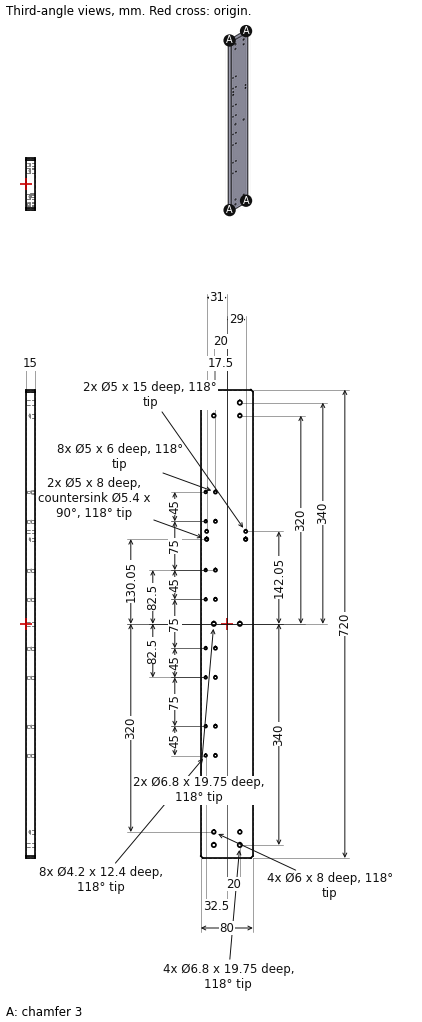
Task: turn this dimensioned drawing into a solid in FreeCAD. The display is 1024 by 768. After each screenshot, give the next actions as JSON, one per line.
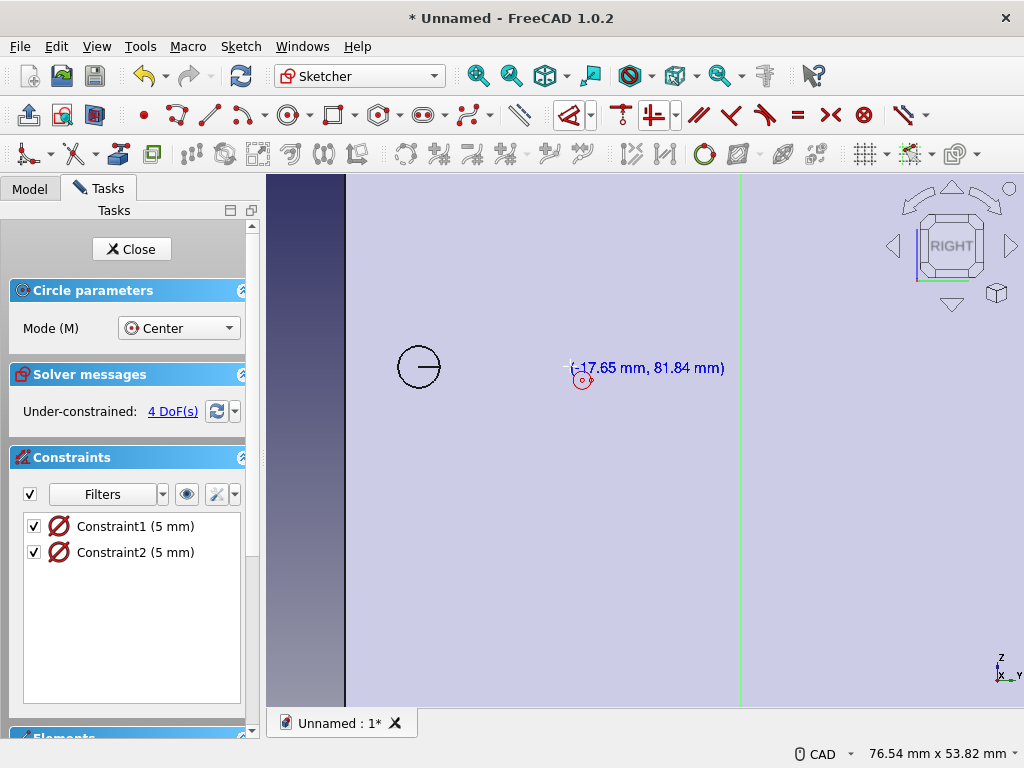
{"action": "scroll", "coordinate": [570, 366], "scroll_direction": "down", "scroll_amount": 12}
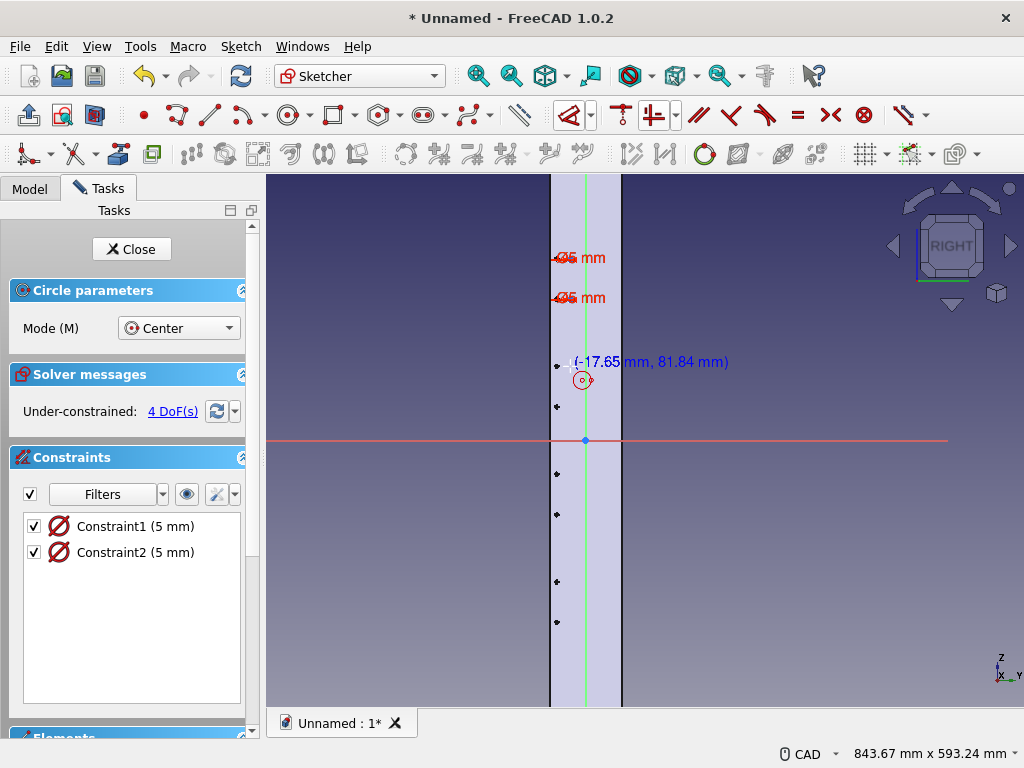
{"action": "left_click", "coordinate": [570, 366]}
{"action": "mouse_move", "coordinate": [572, 365]}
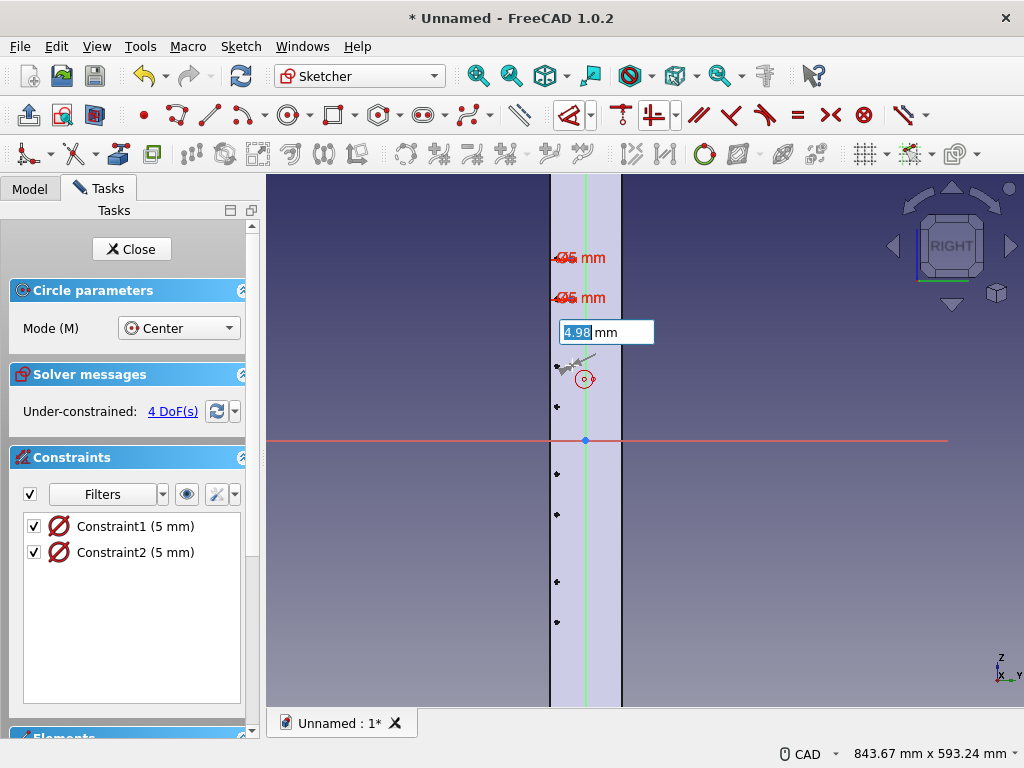
{"action": "type", "text": "5"}
{"action": "key", "text": "Return"}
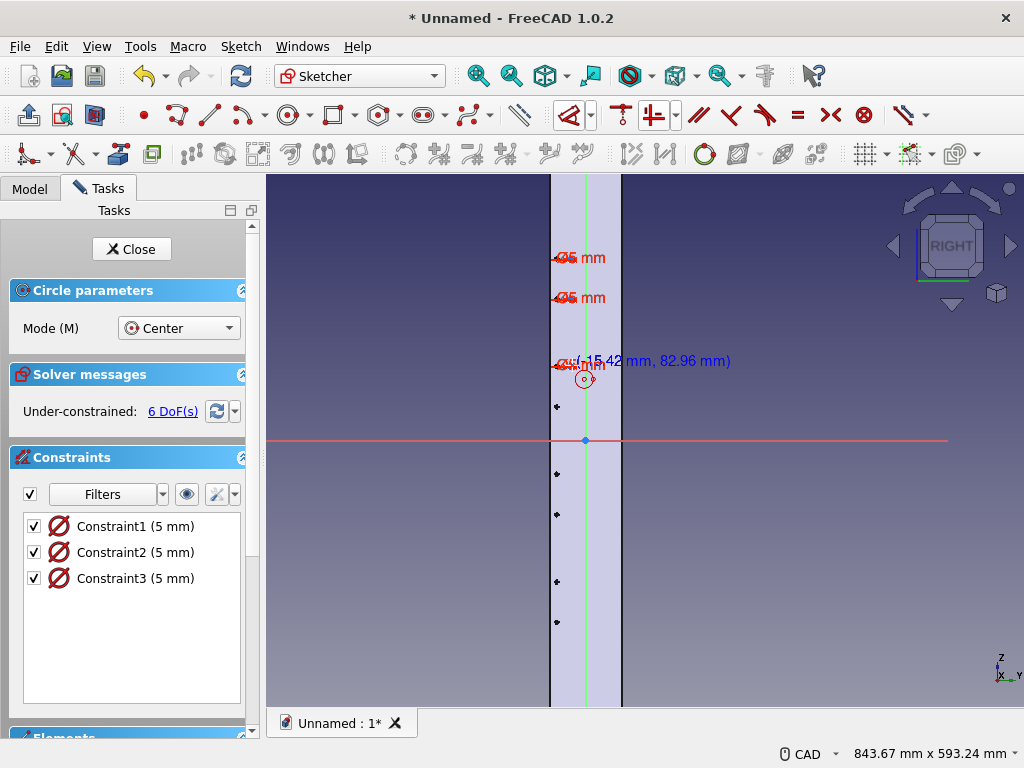
{"action": "scroll", "coordinate": [570, 407], "scroll_direction": "up", "scroll_amount": 12}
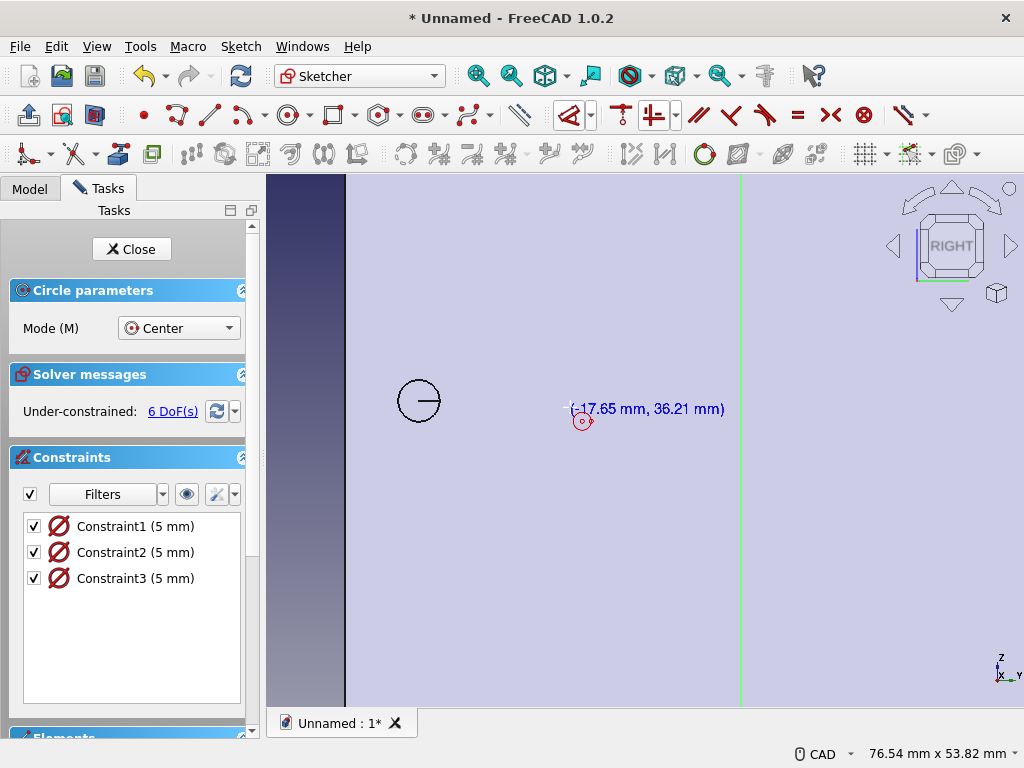
{"action": "scroll", "coordinate": [570, 407], "scroll_direction": "down", "scroll_amount": 12}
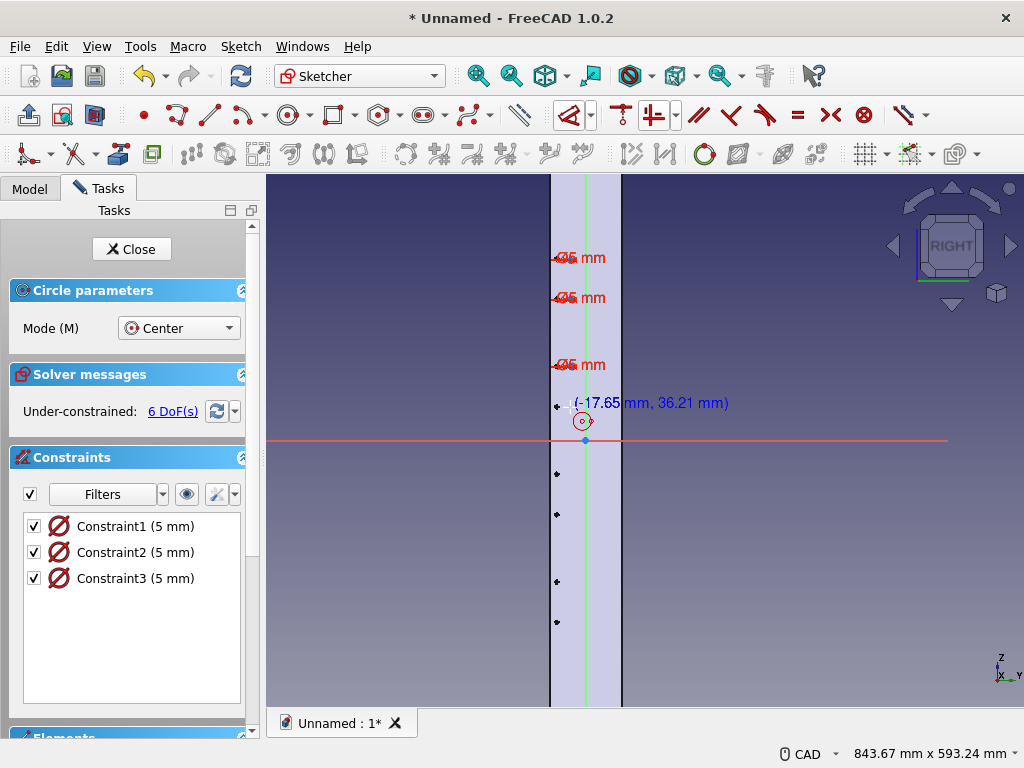
{"action": "left_click", "coordinate": [570, 407]}
{"action": "mouse_move", "coordinate": [572, 405]}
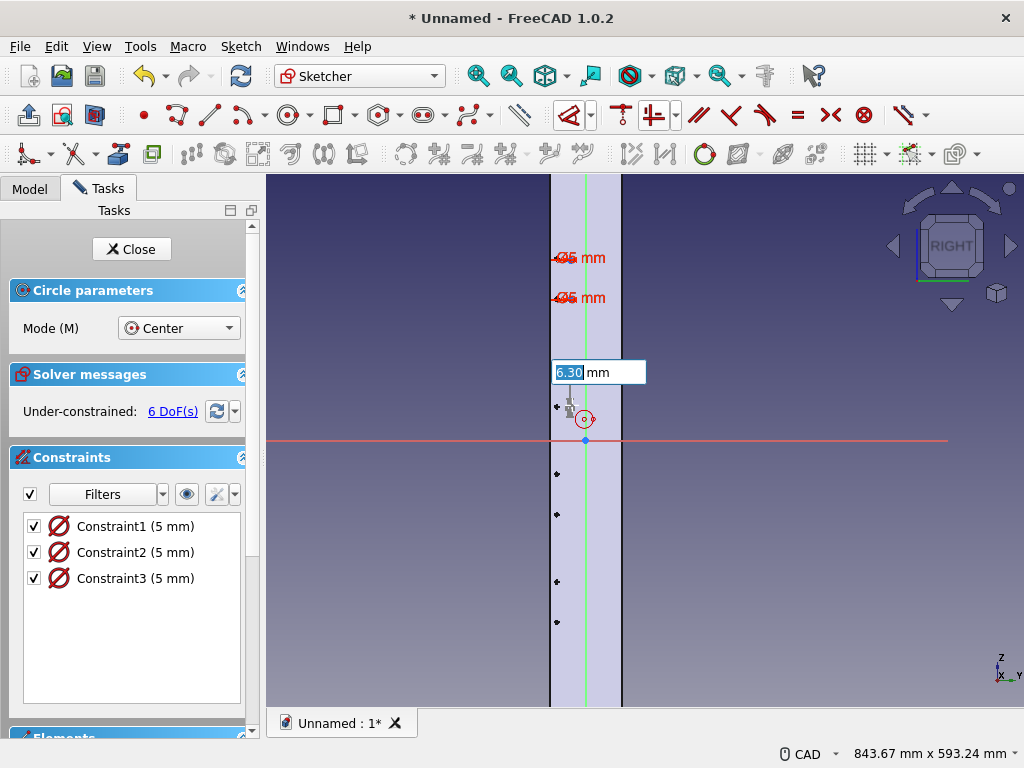
{"action": "type", "text": "5"}
{"action": "key", "text": "Return"}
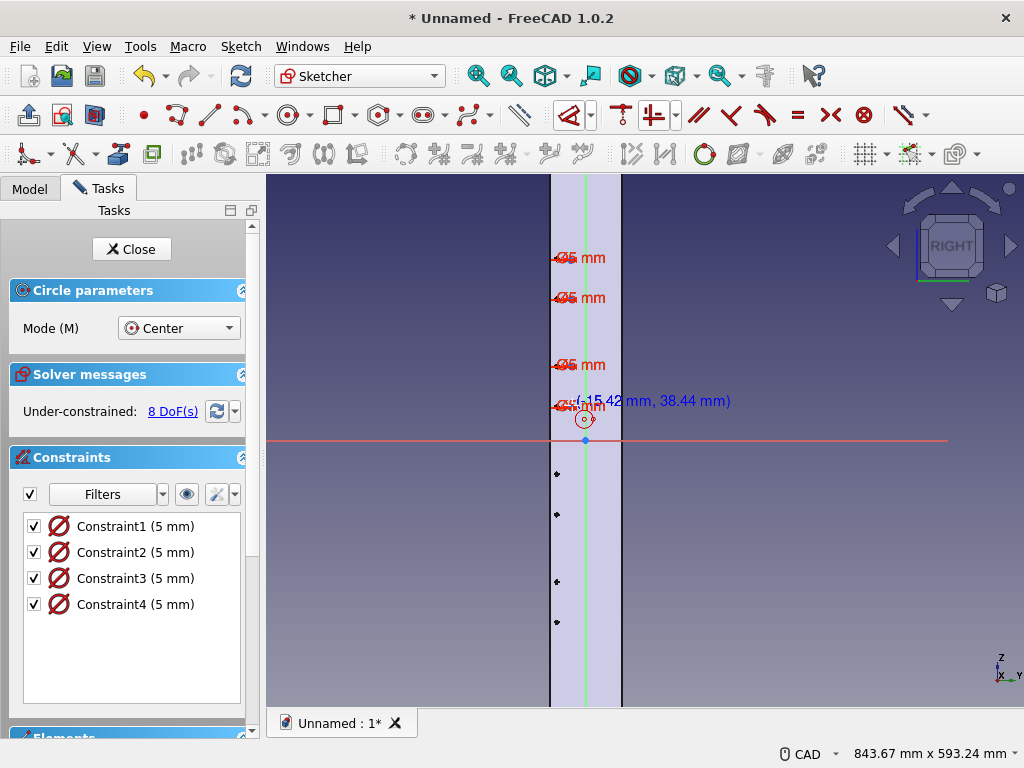
{"action": "scroll", "coordinate": [570, 474], "scroll_direction": "up", "scroll_amount": 12}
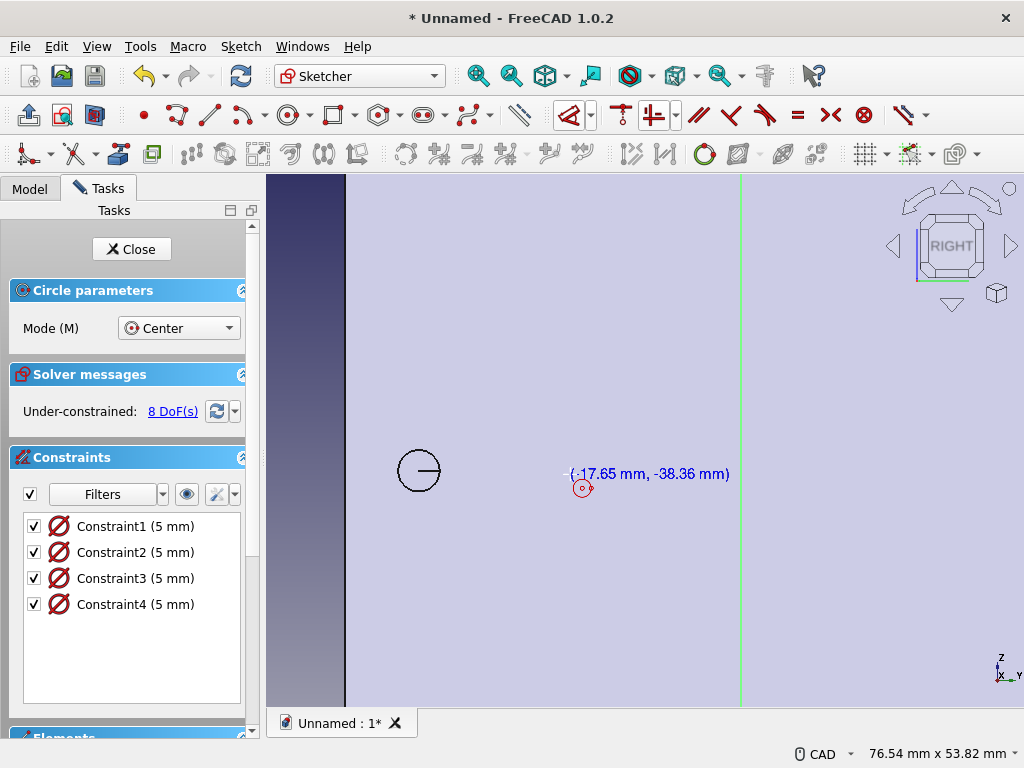
{"action": "scroll", "coordinate": [570, 475], "scroll_direction": "down", "scroll_amount": 12}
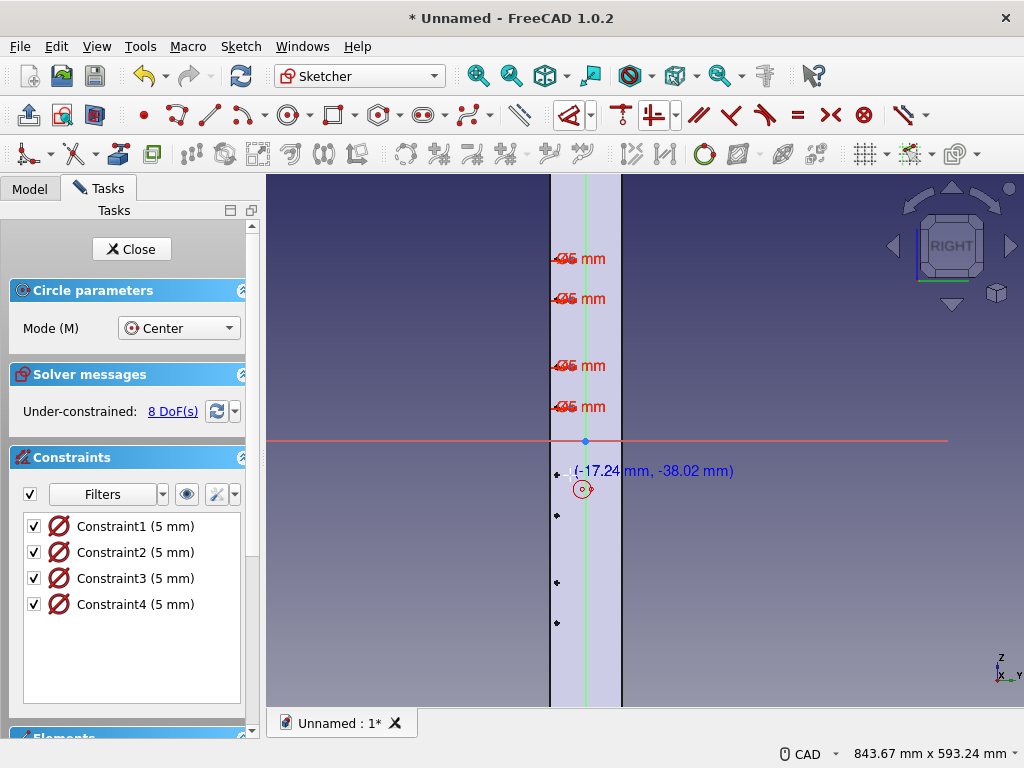
{"action": "left_click", "coordinate": [570, 475]}
{"action": "mouse_move", "coordinate": [572, 474]}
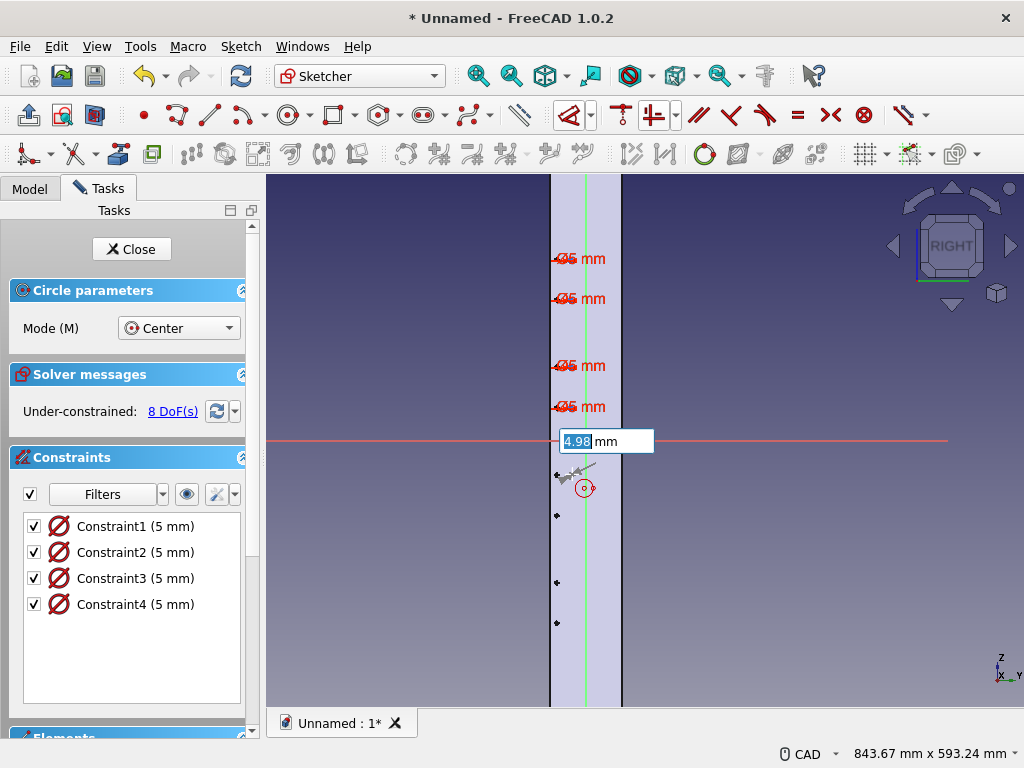
{"action": "type", "text": "5"}
{"action": "key", "text": "Return"}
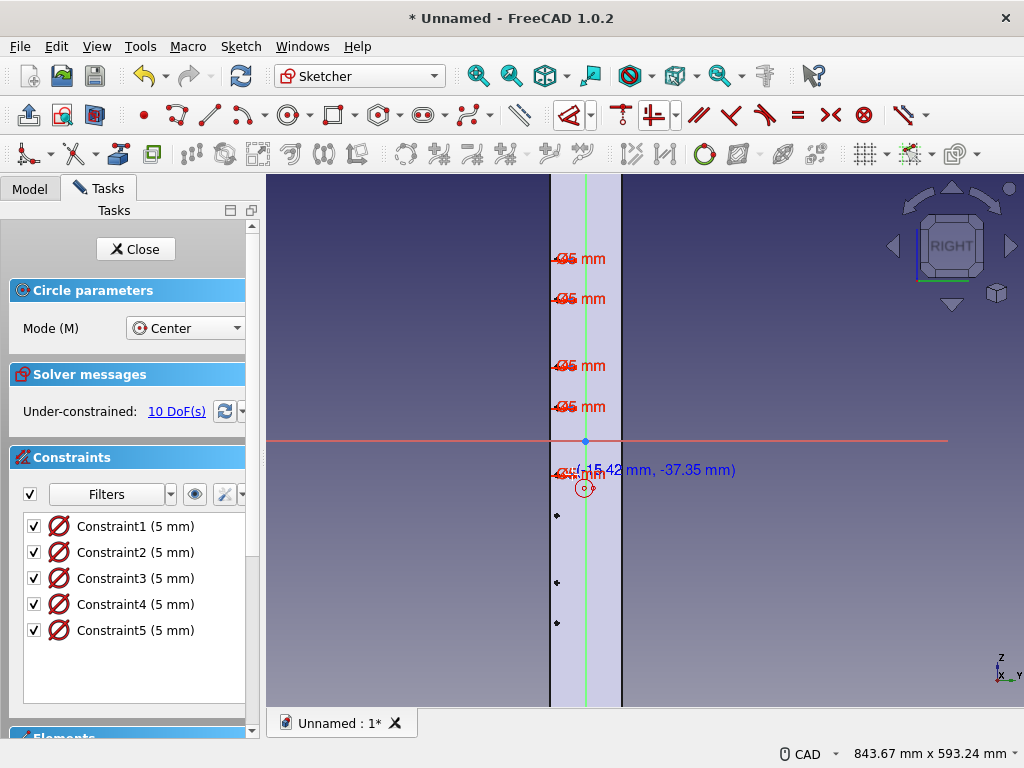
{"action": "scroll", "coordinate": [570, 516], "scroll_direction": "up", "scroll_amount": 12}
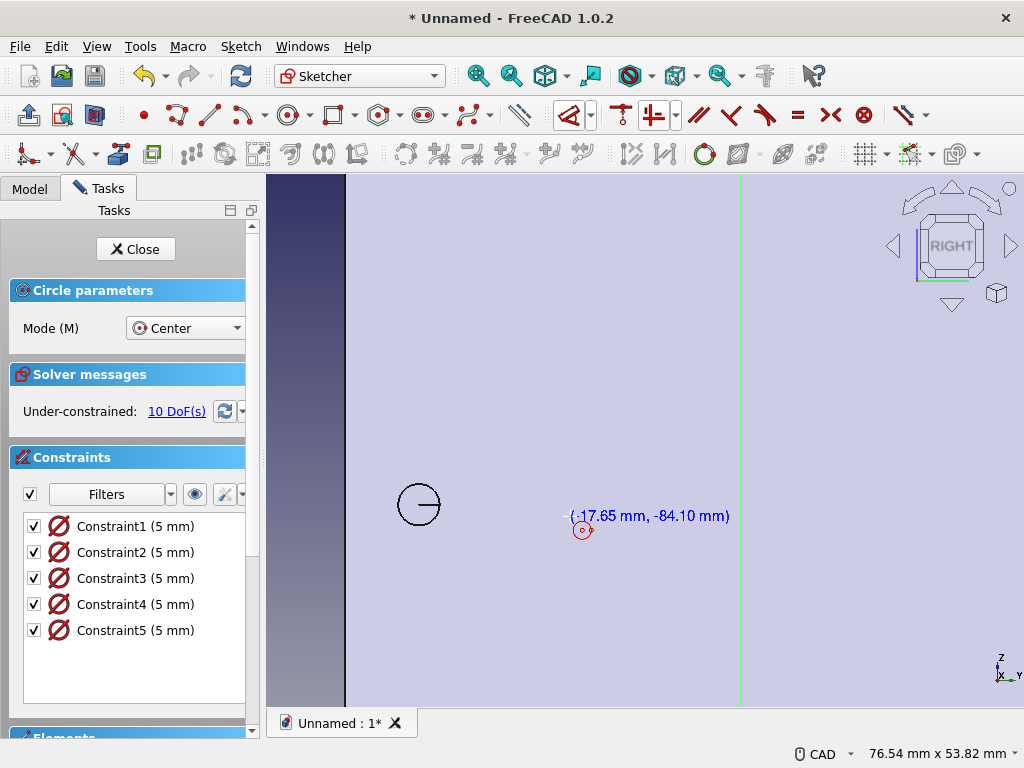
{"action": "scroll", "coordinate": [570, 516], "scroll_direction": "down", "scroll_amount": 12}